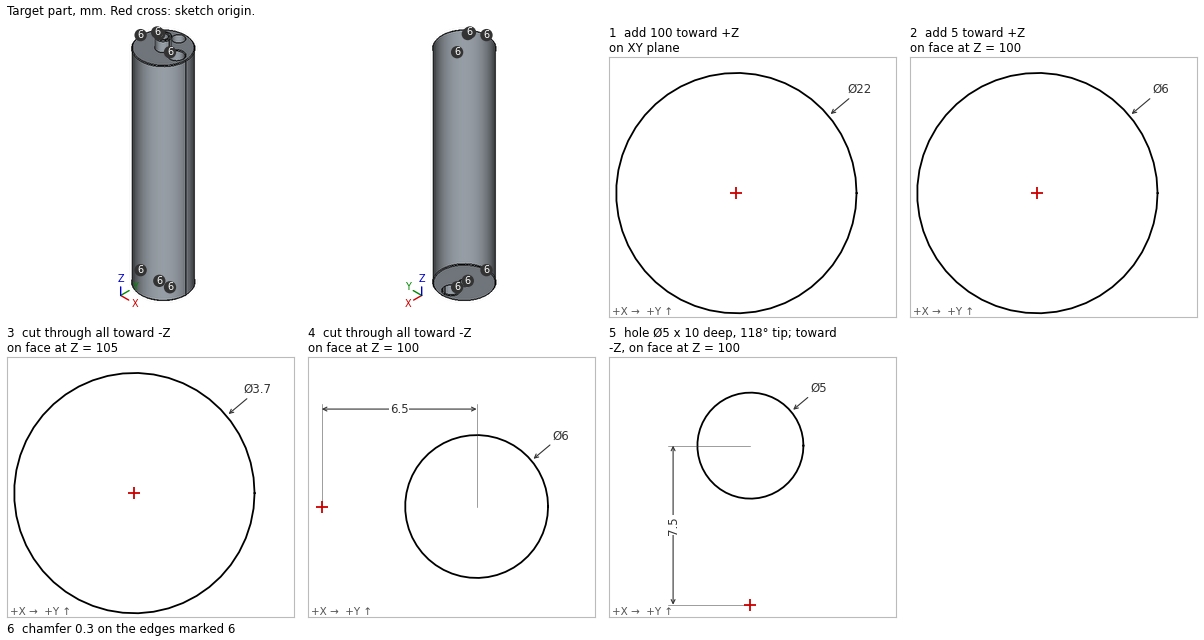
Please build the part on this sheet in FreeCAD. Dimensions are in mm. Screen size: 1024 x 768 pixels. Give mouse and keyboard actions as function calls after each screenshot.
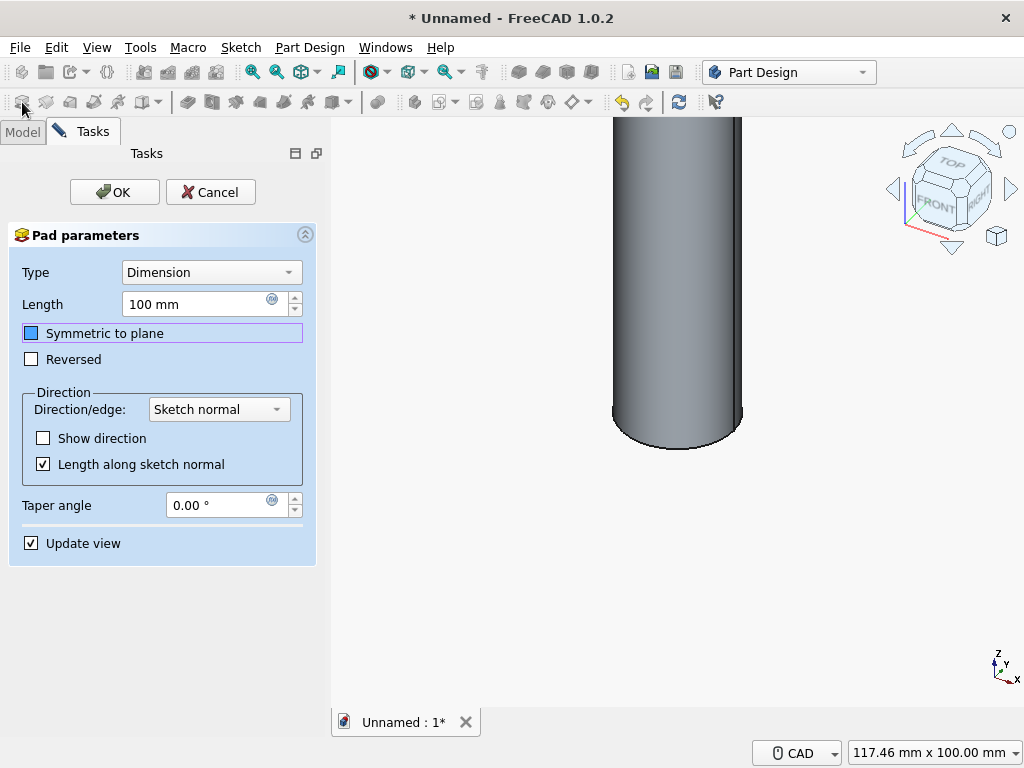
click(115, 192)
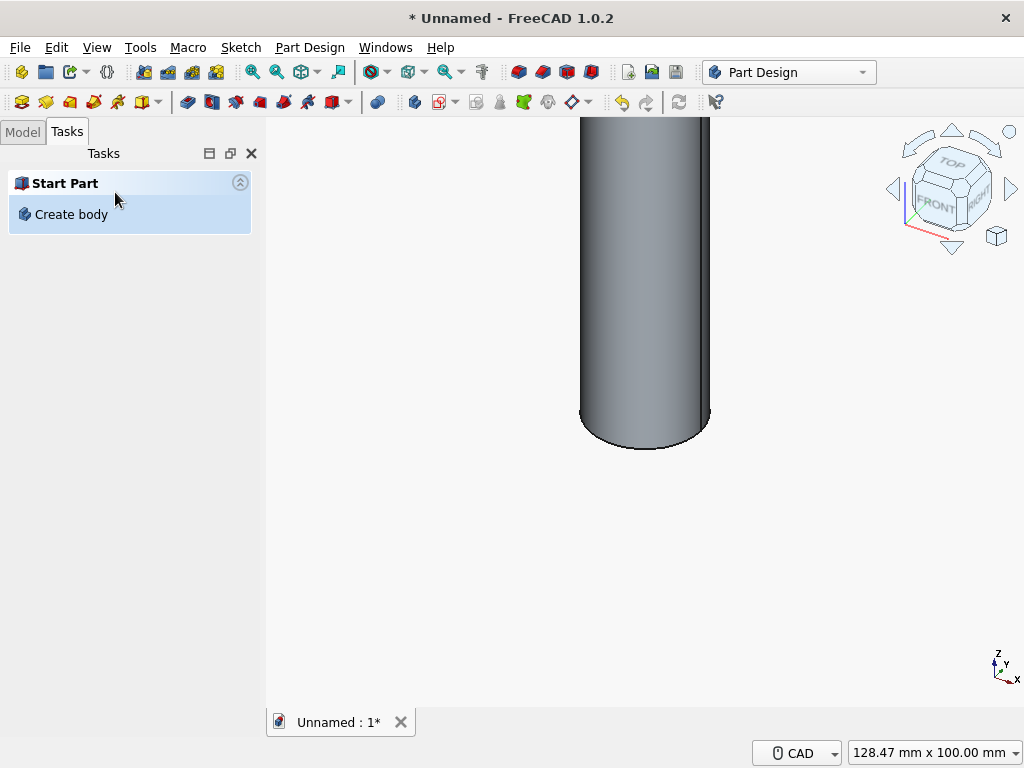
key(v)
key(f)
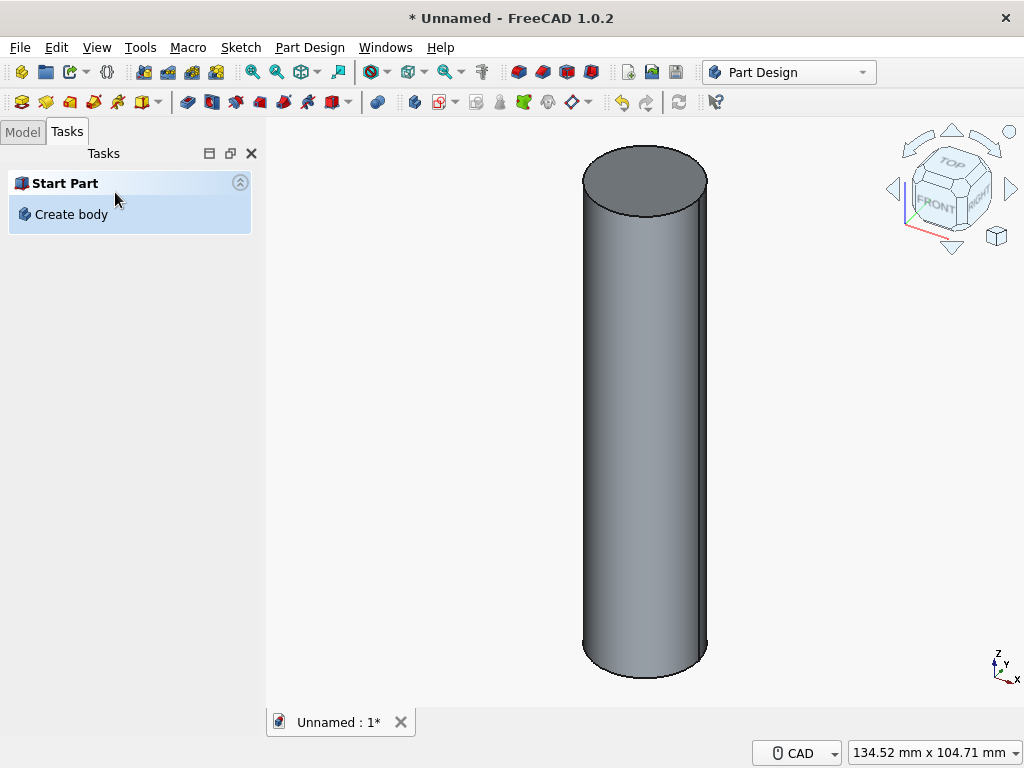
click(645, 180)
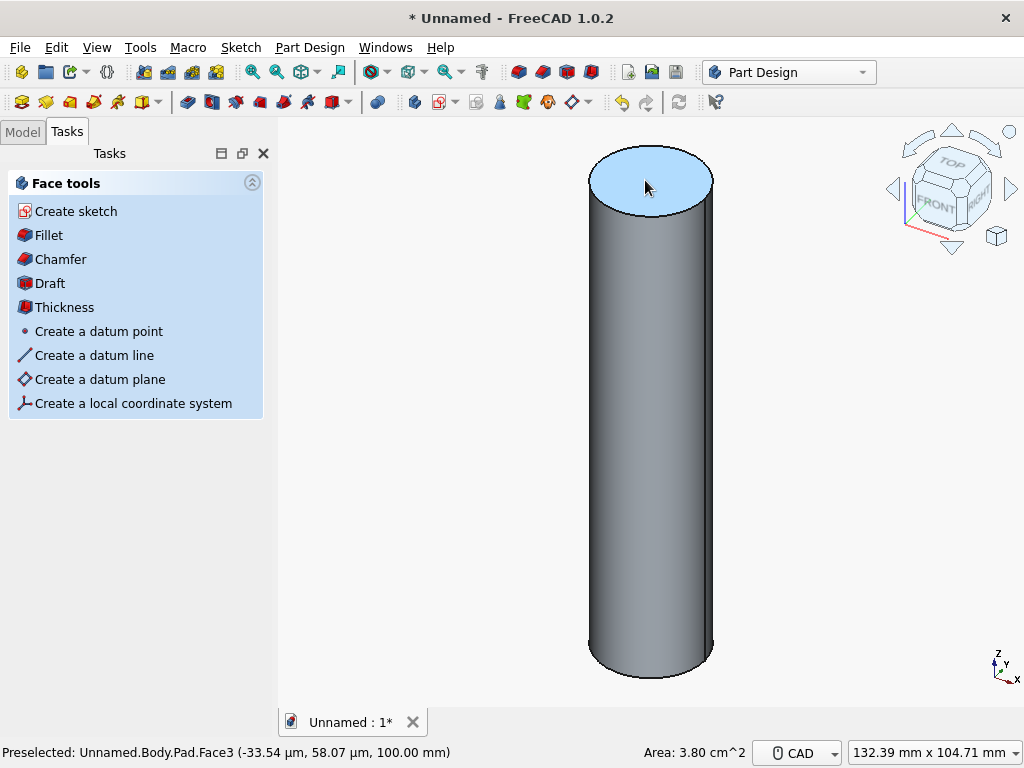
click(440, 102)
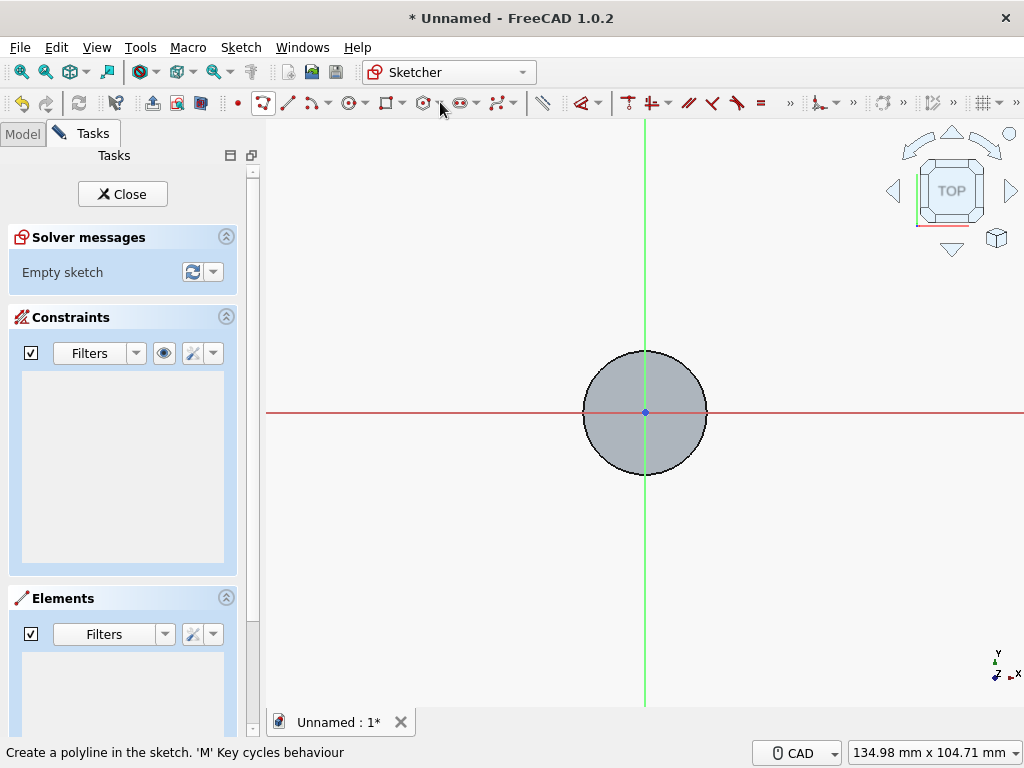
scroll(652, 413, up, 12)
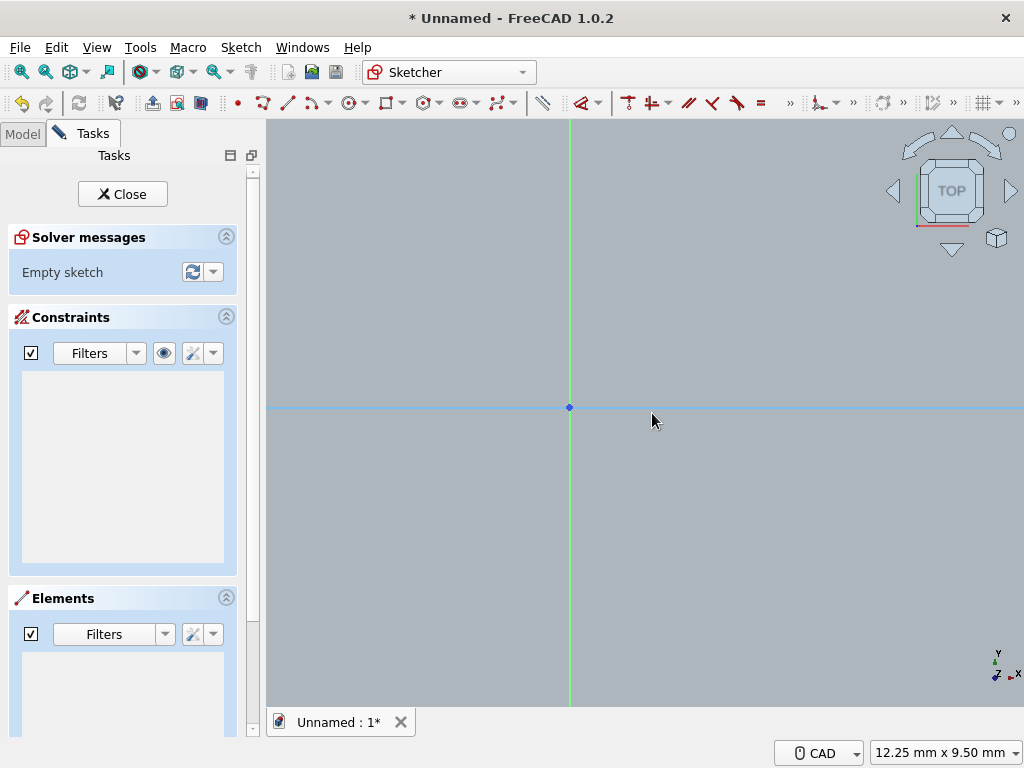
click(350, 104)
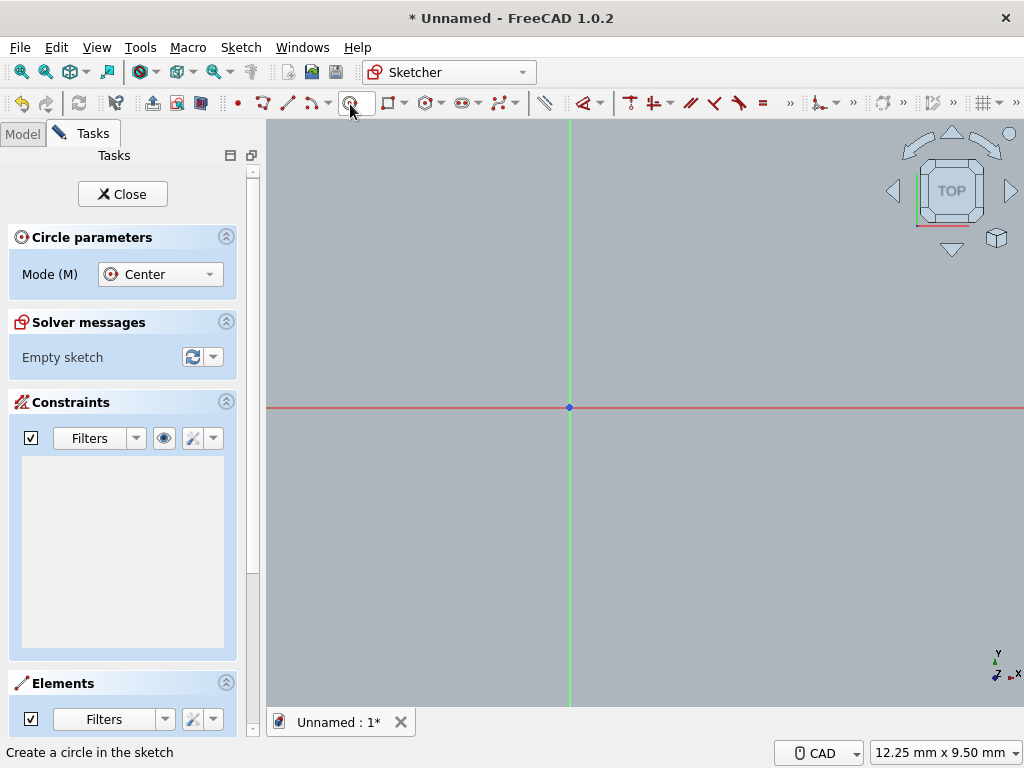
click(570, 408)
click(701, 277)
key(Escape)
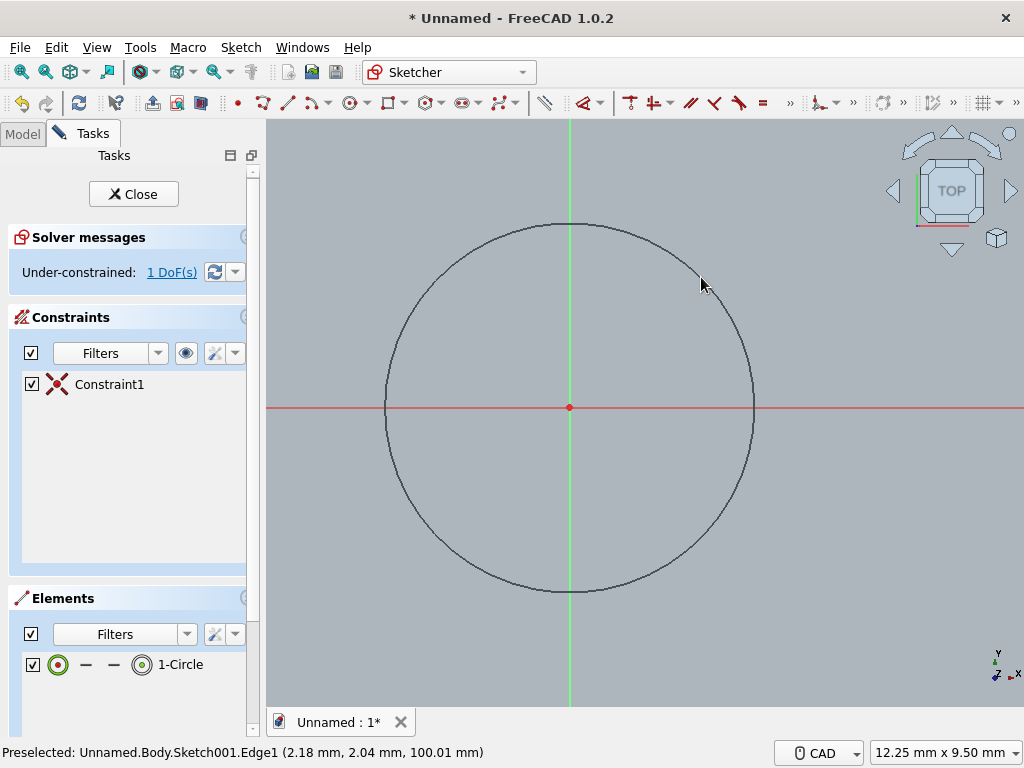
click(700, 277)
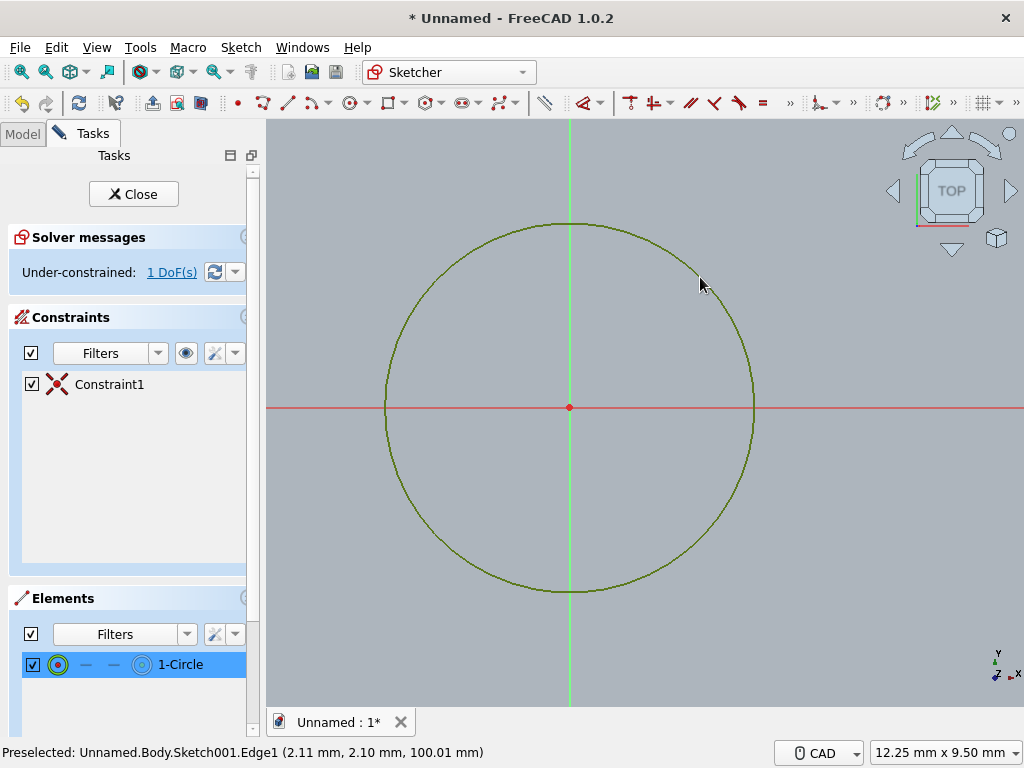
click(602, 104)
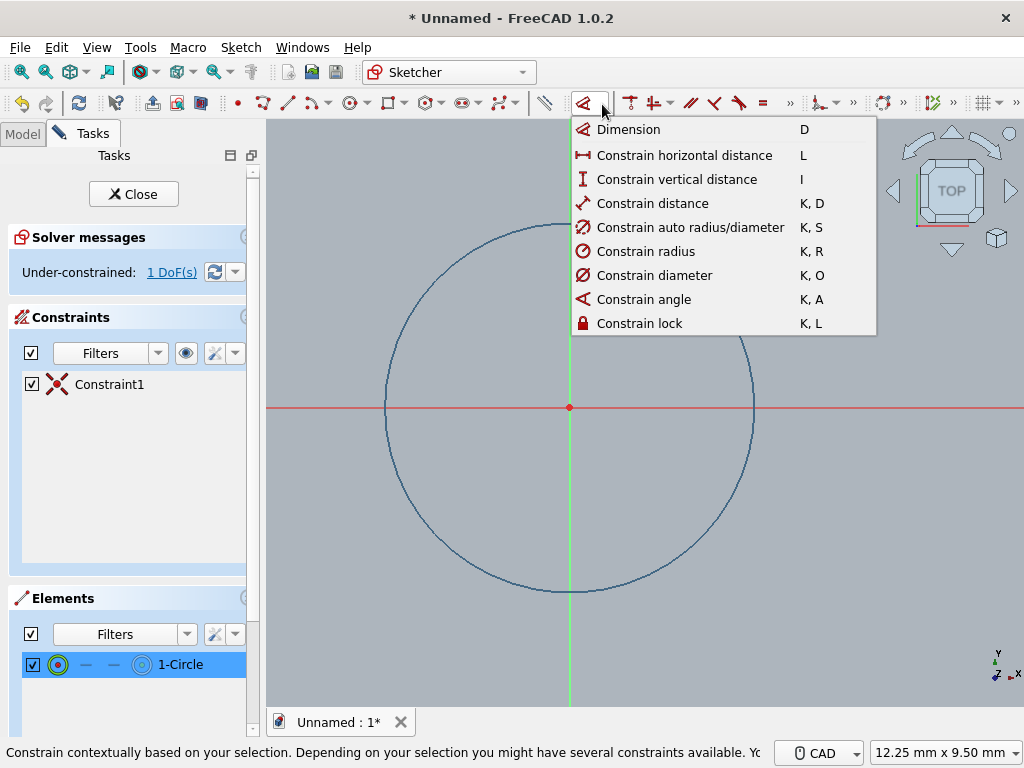
click(724, 275)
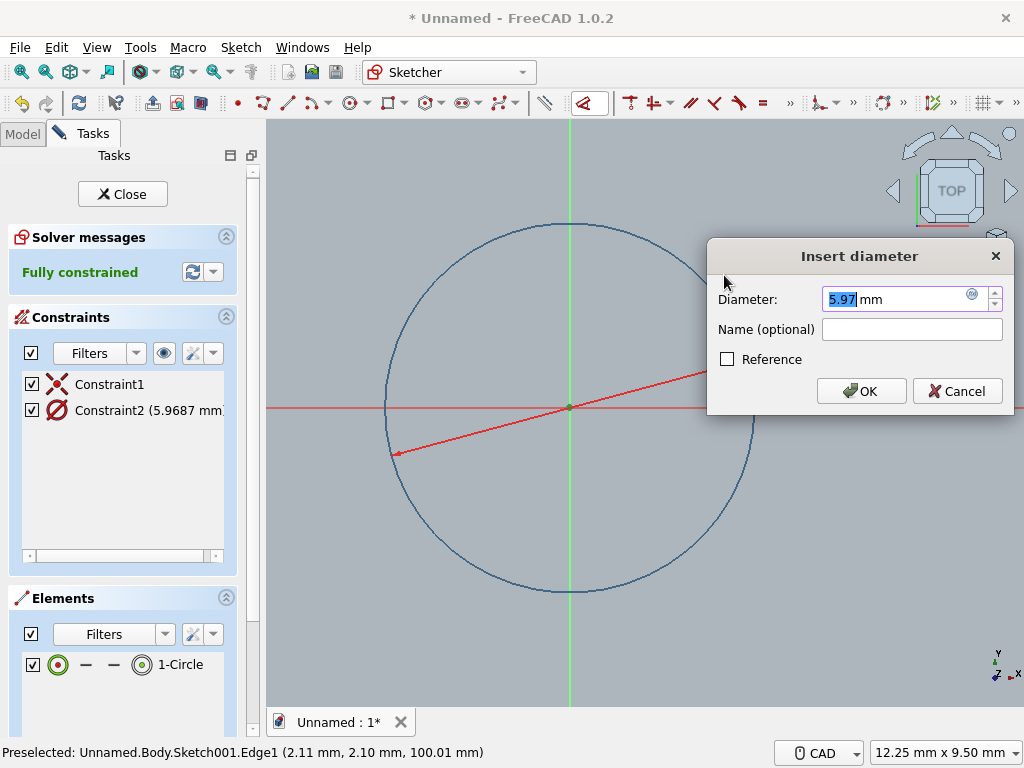
text(6)
key(Return)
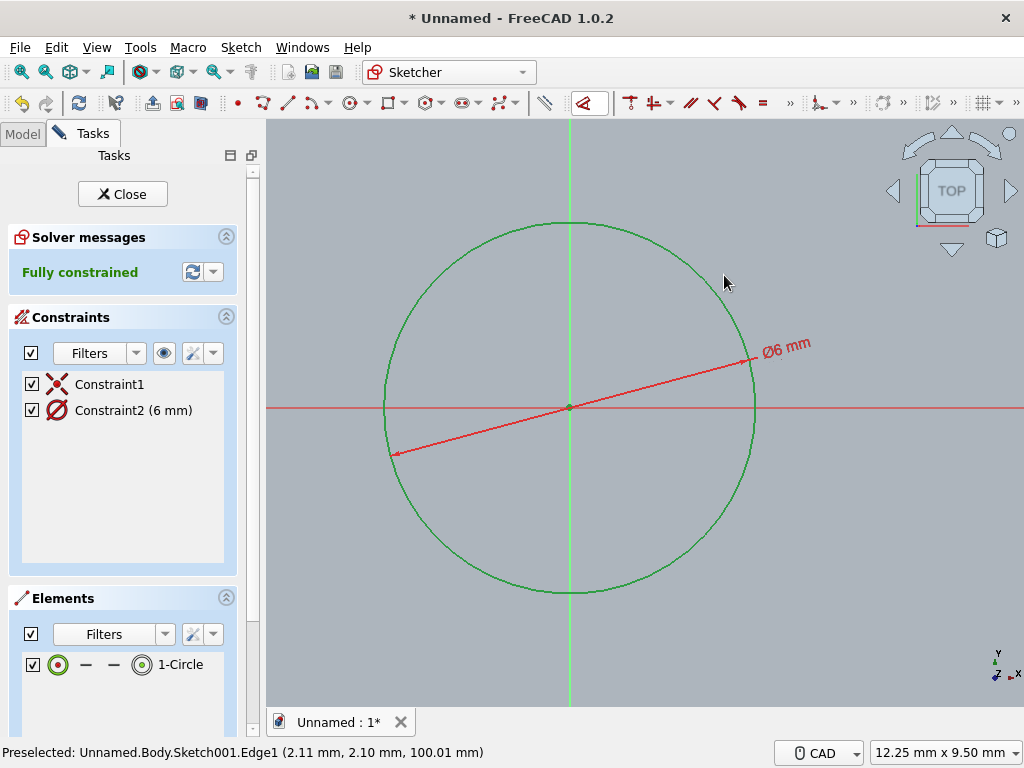
click(123, 194)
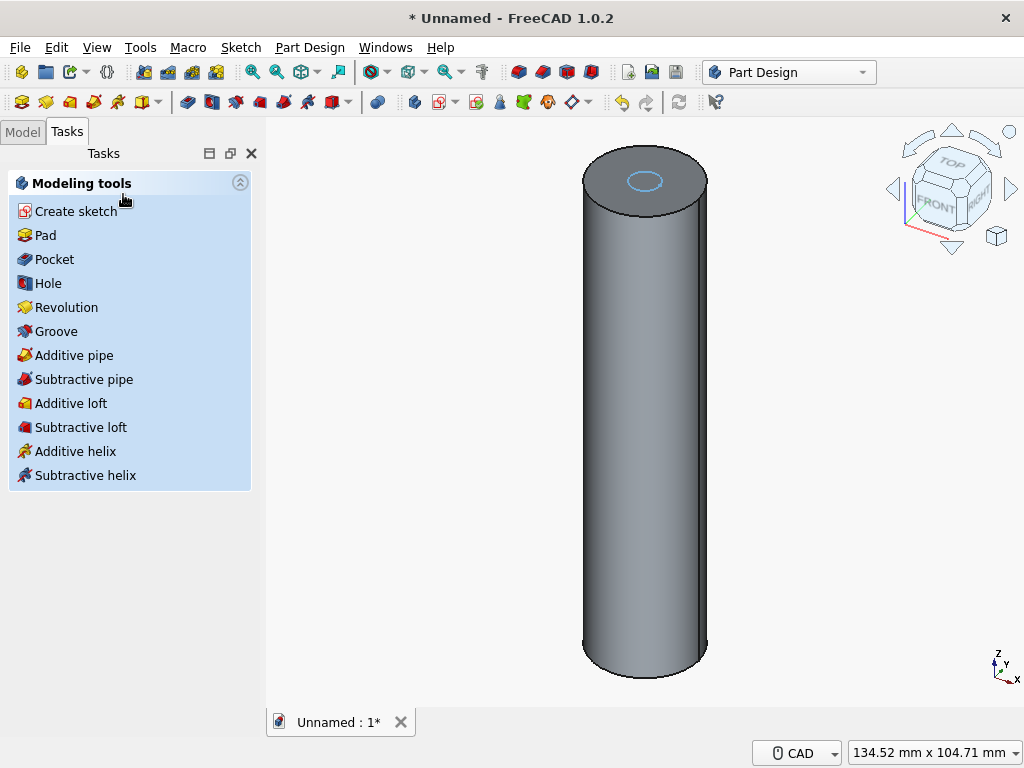
click(22, 102)